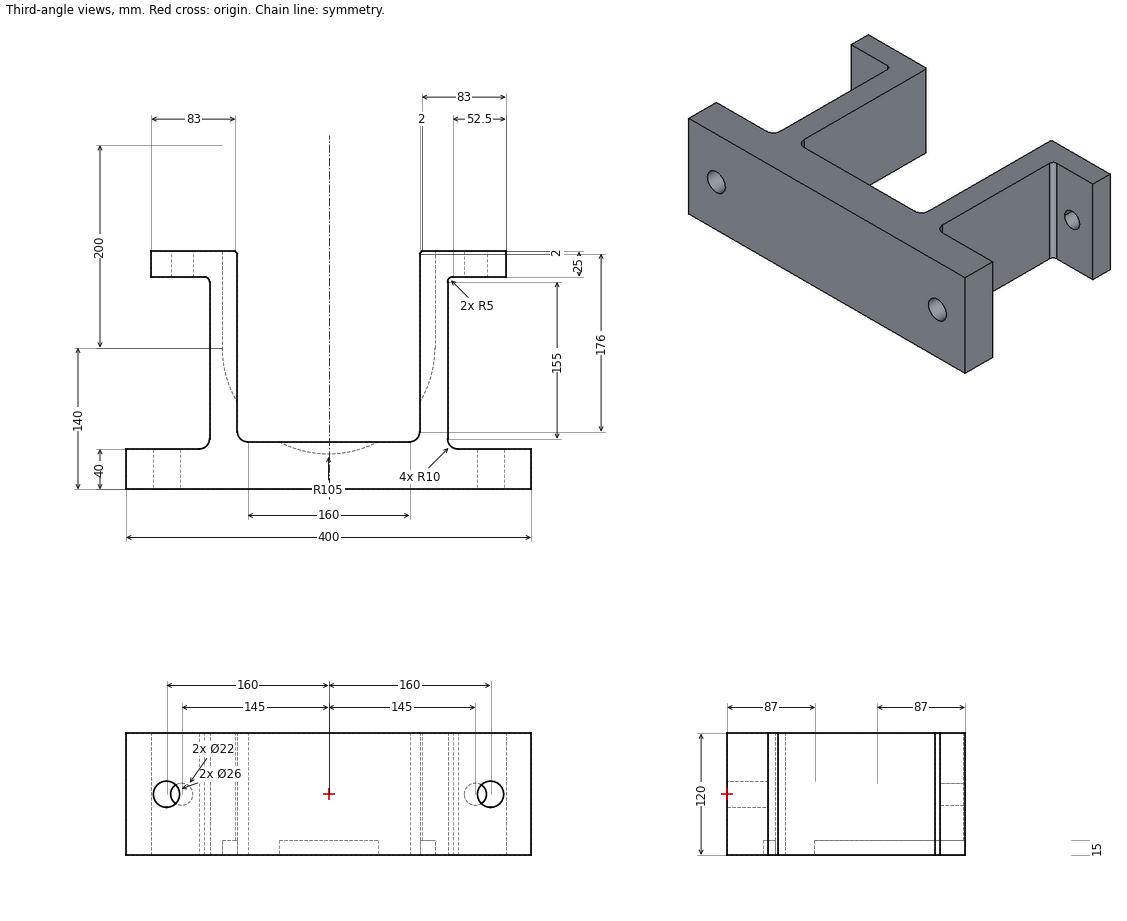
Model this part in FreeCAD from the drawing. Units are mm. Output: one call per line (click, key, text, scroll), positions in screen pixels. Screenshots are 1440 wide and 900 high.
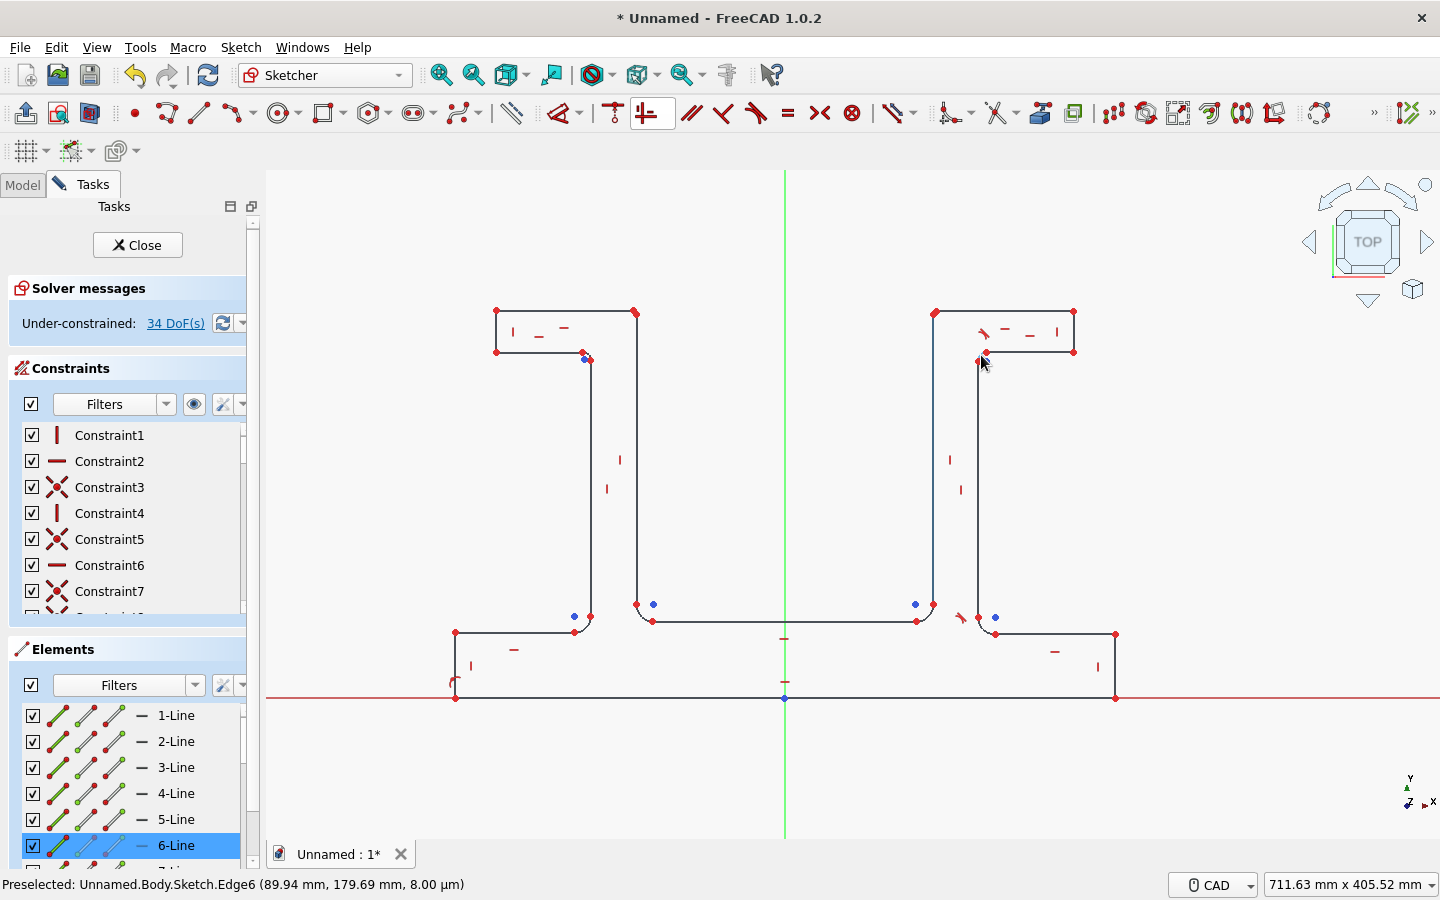
scroll(924, 620, up, 3)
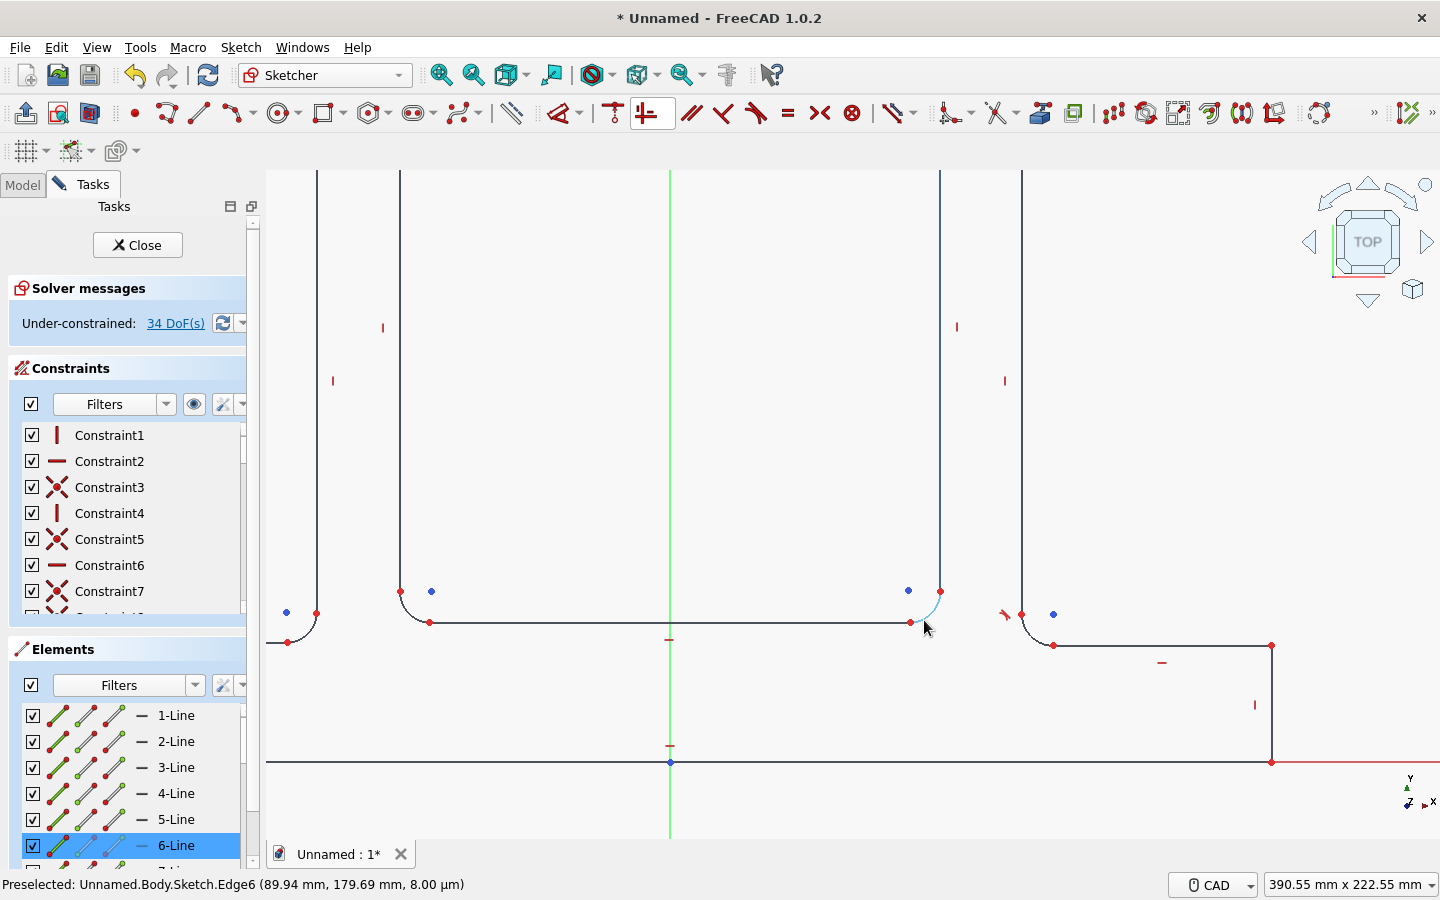
click(924, 619)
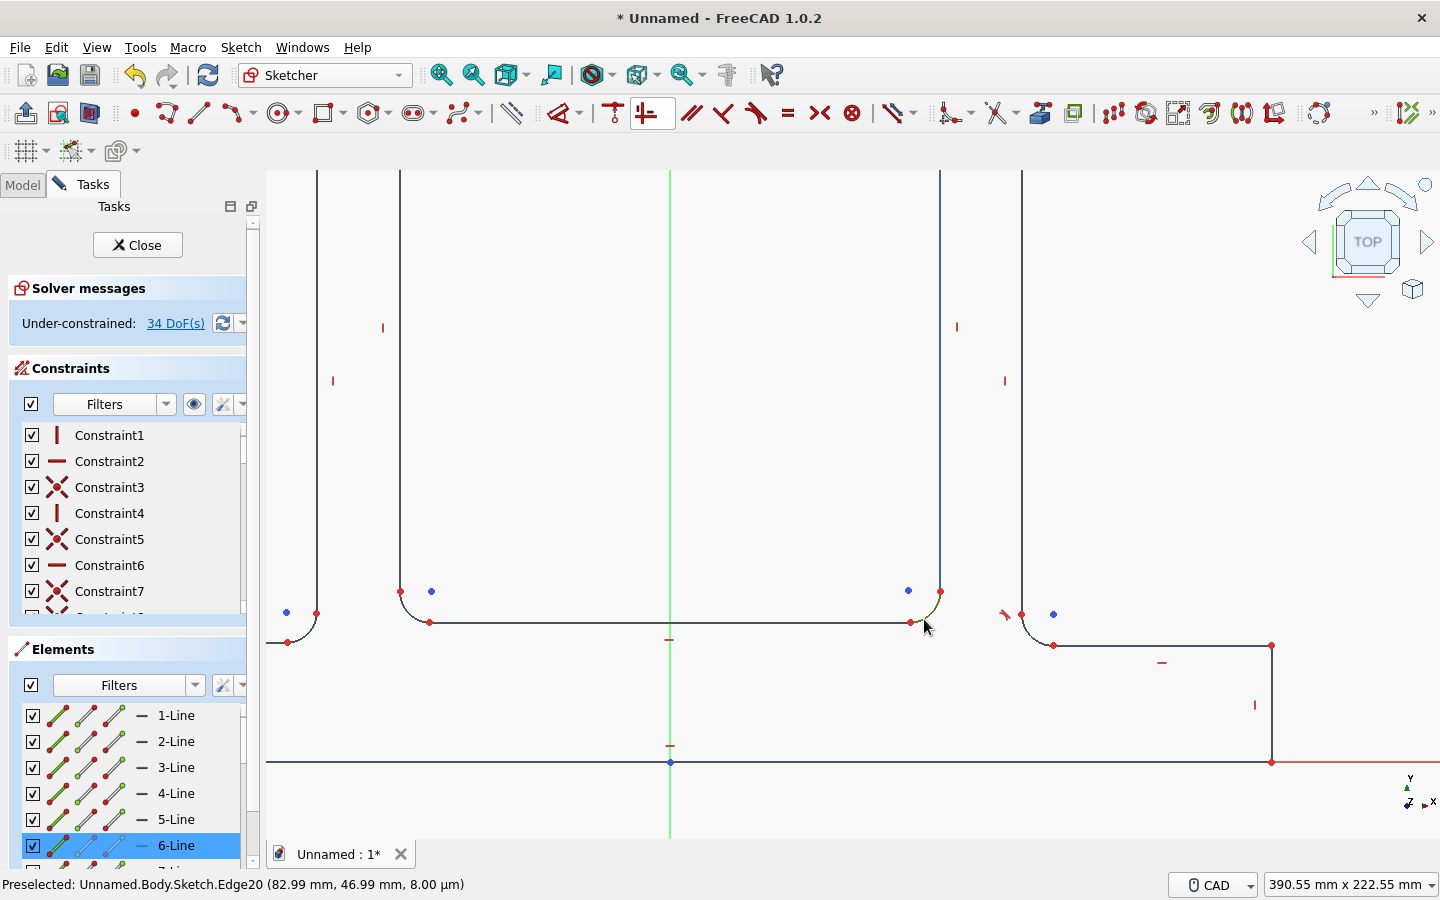
click(756, 114)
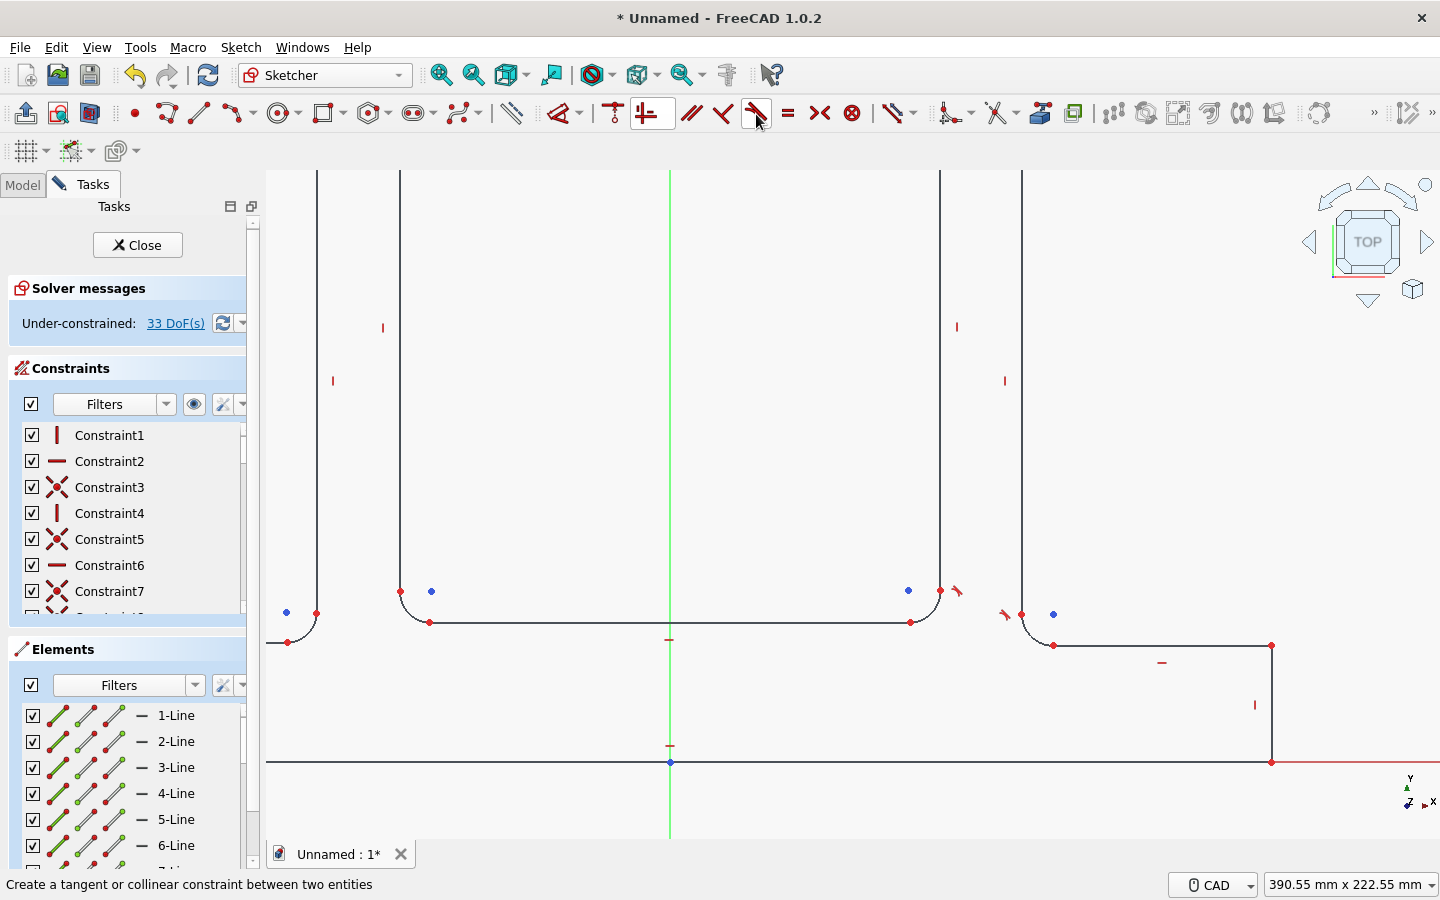
click(766, 623)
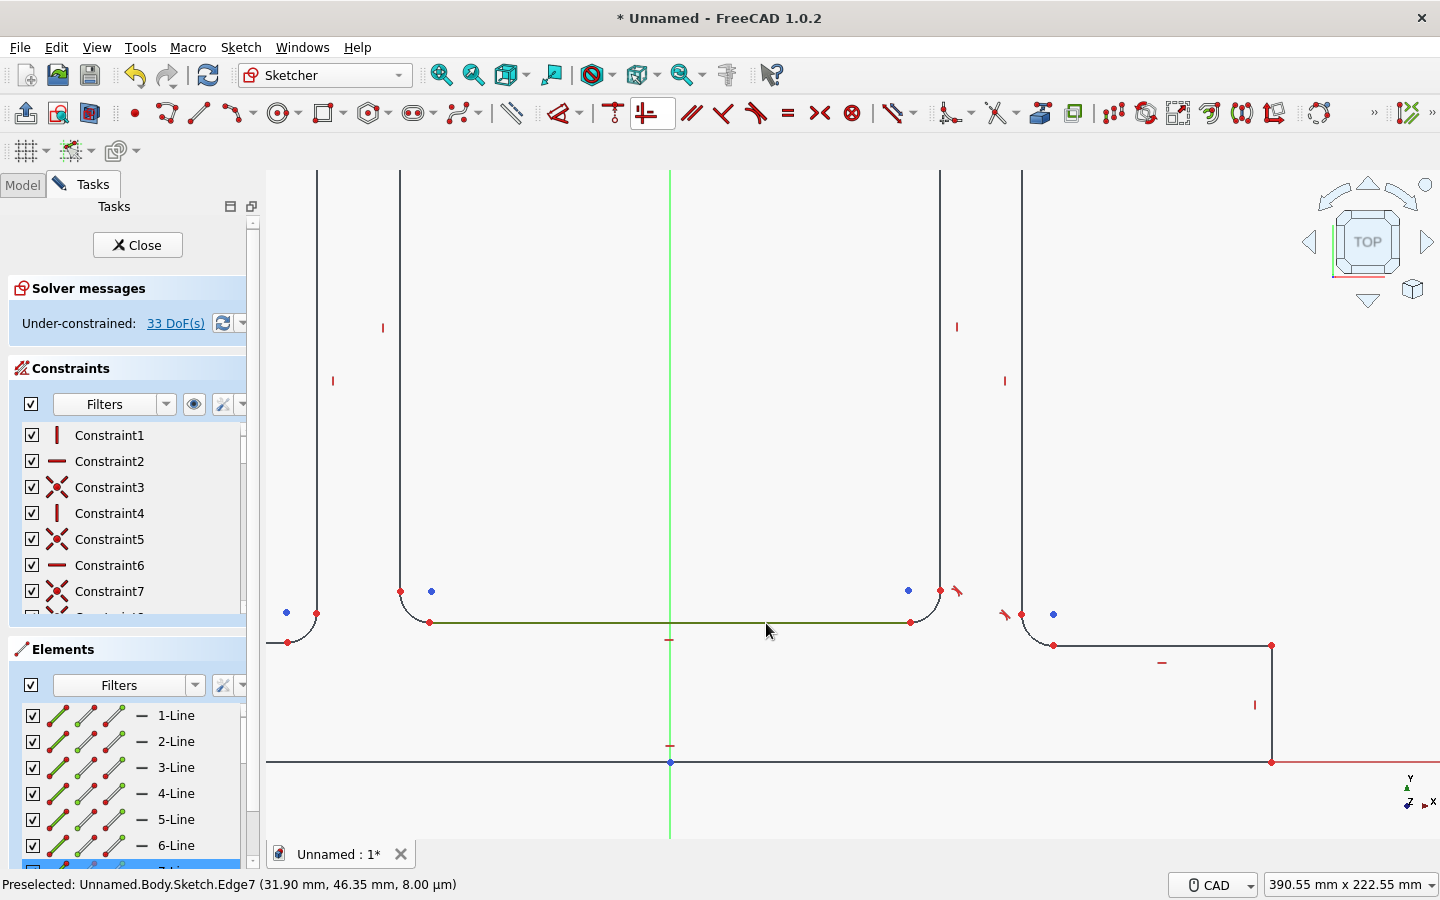
click(924, 619)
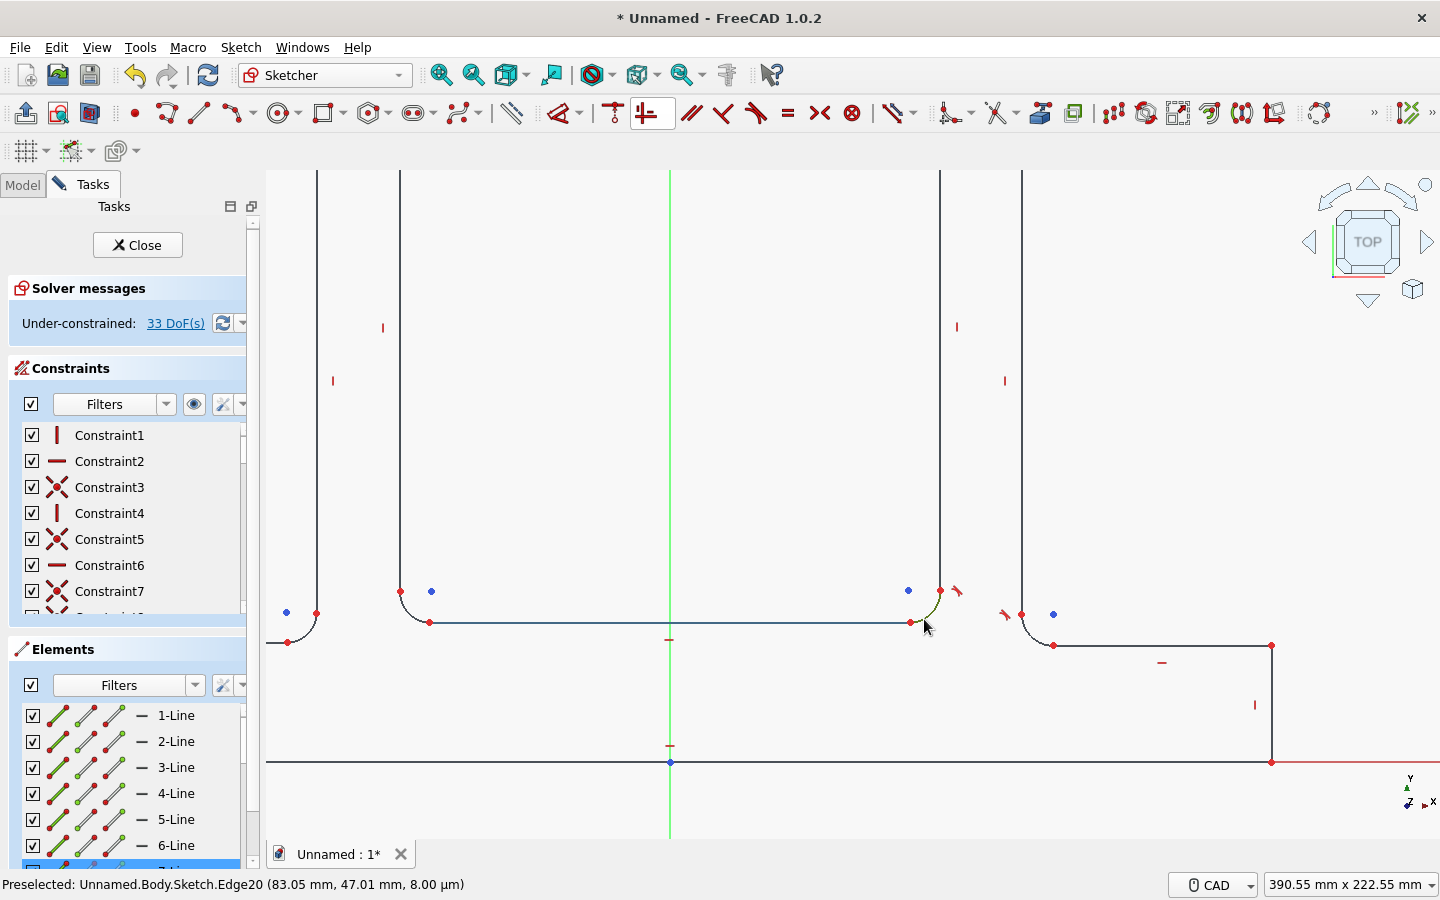
click(756, 114)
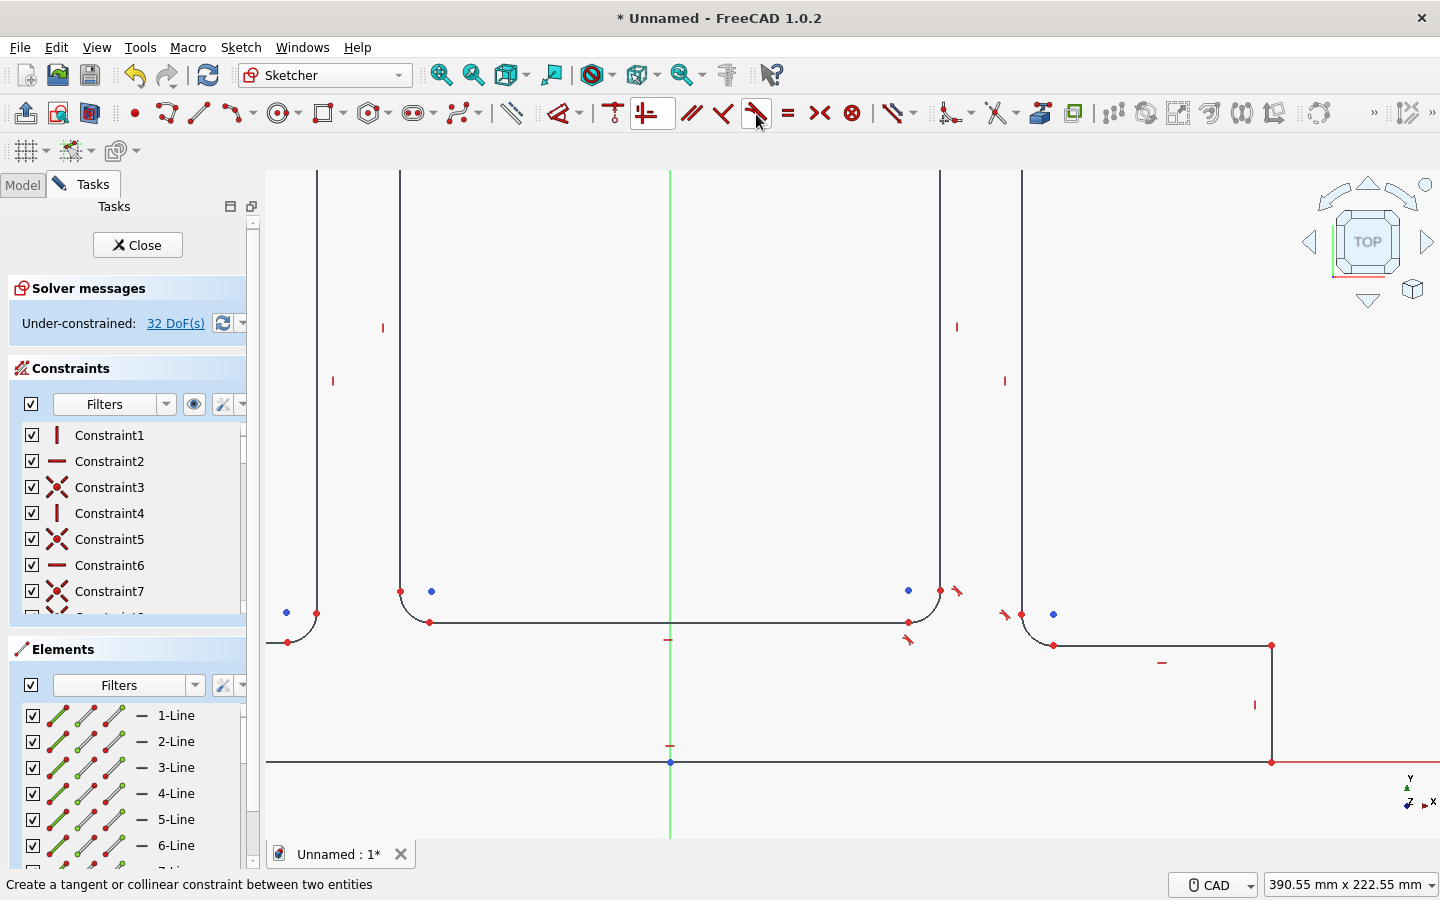
click(765, 623)